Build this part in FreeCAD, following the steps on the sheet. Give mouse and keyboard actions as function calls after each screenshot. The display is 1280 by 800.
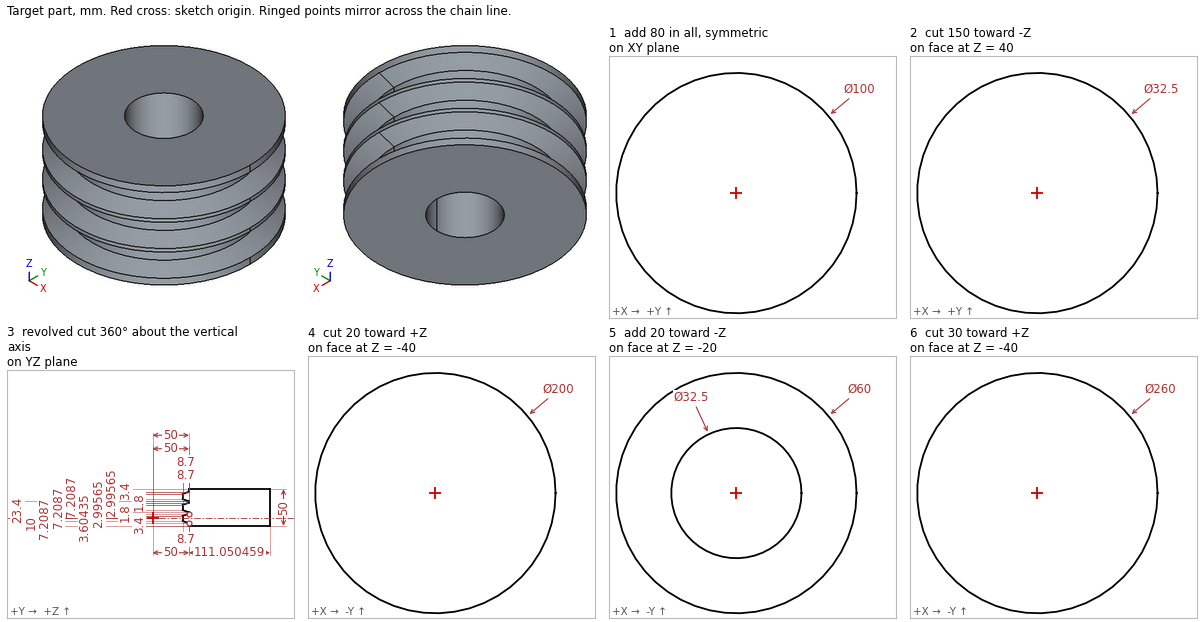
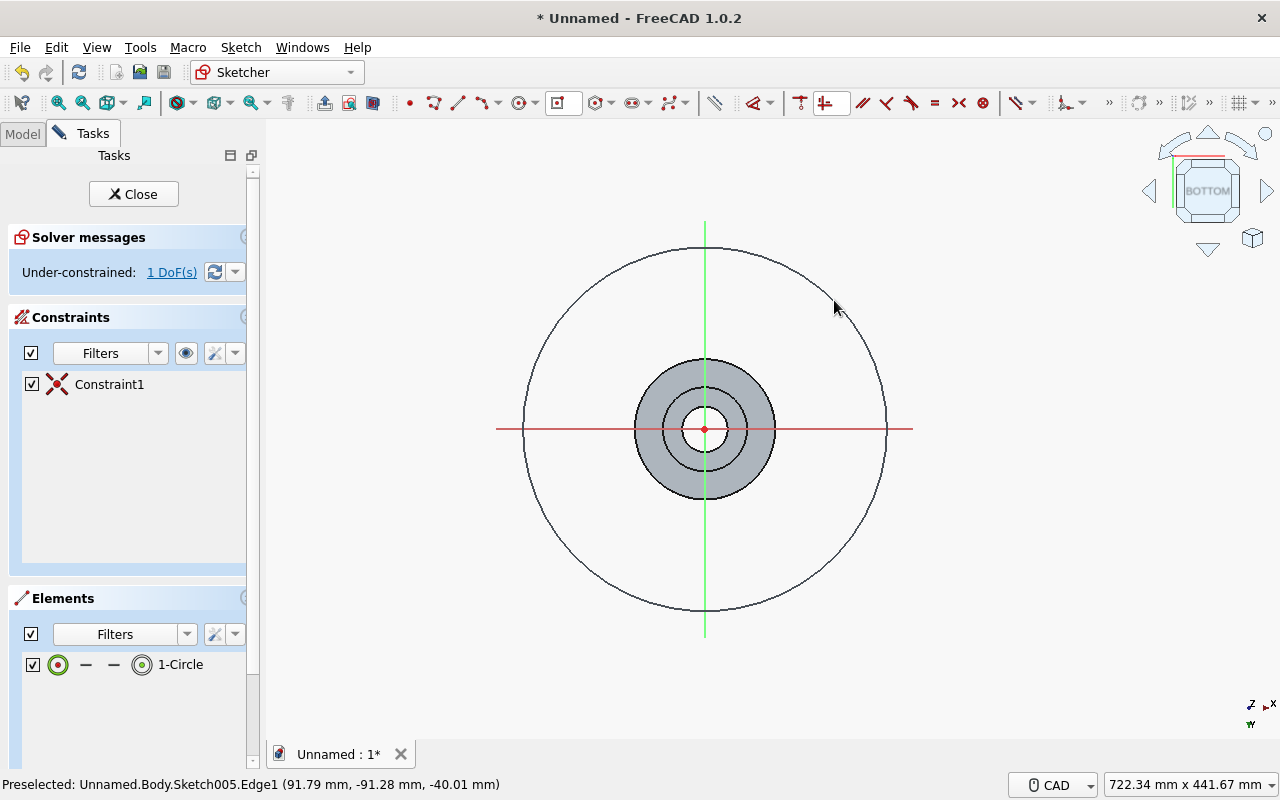
click(754, 104)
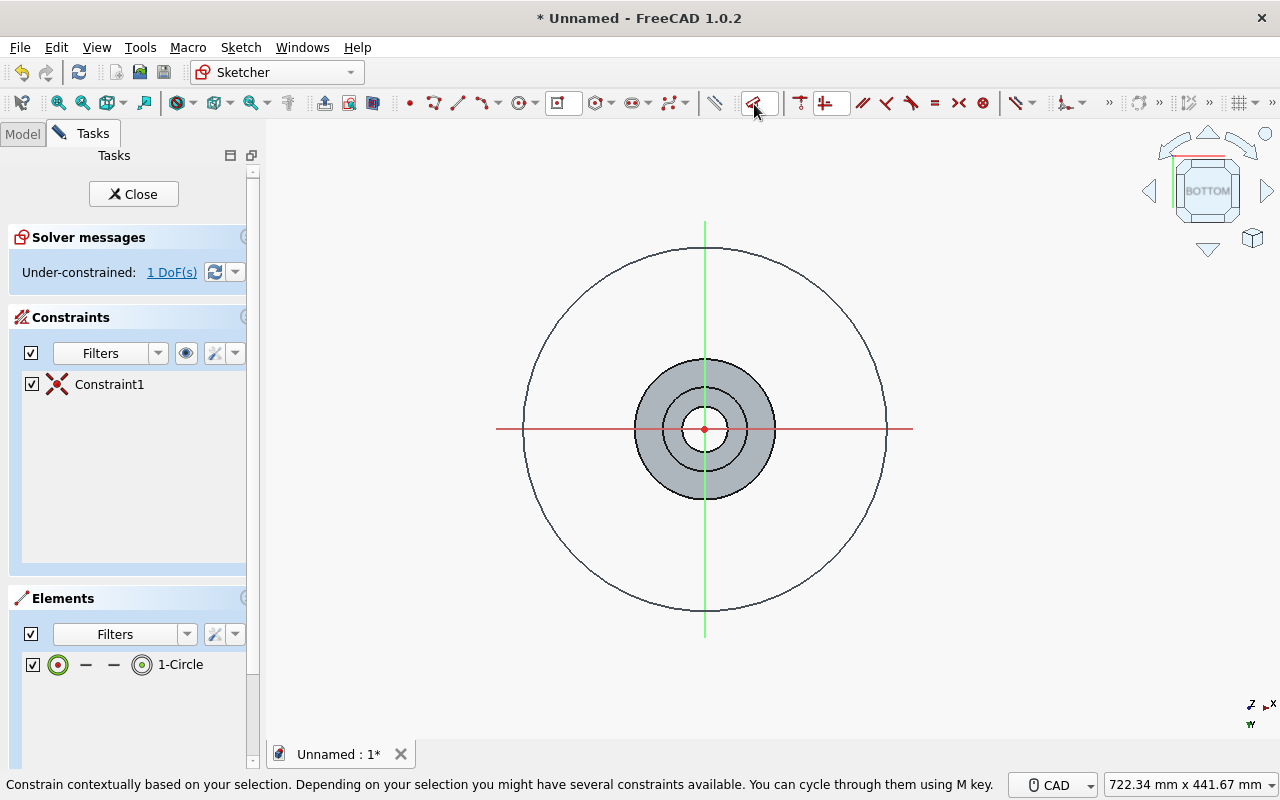
click(833, 300)
click(856, 277)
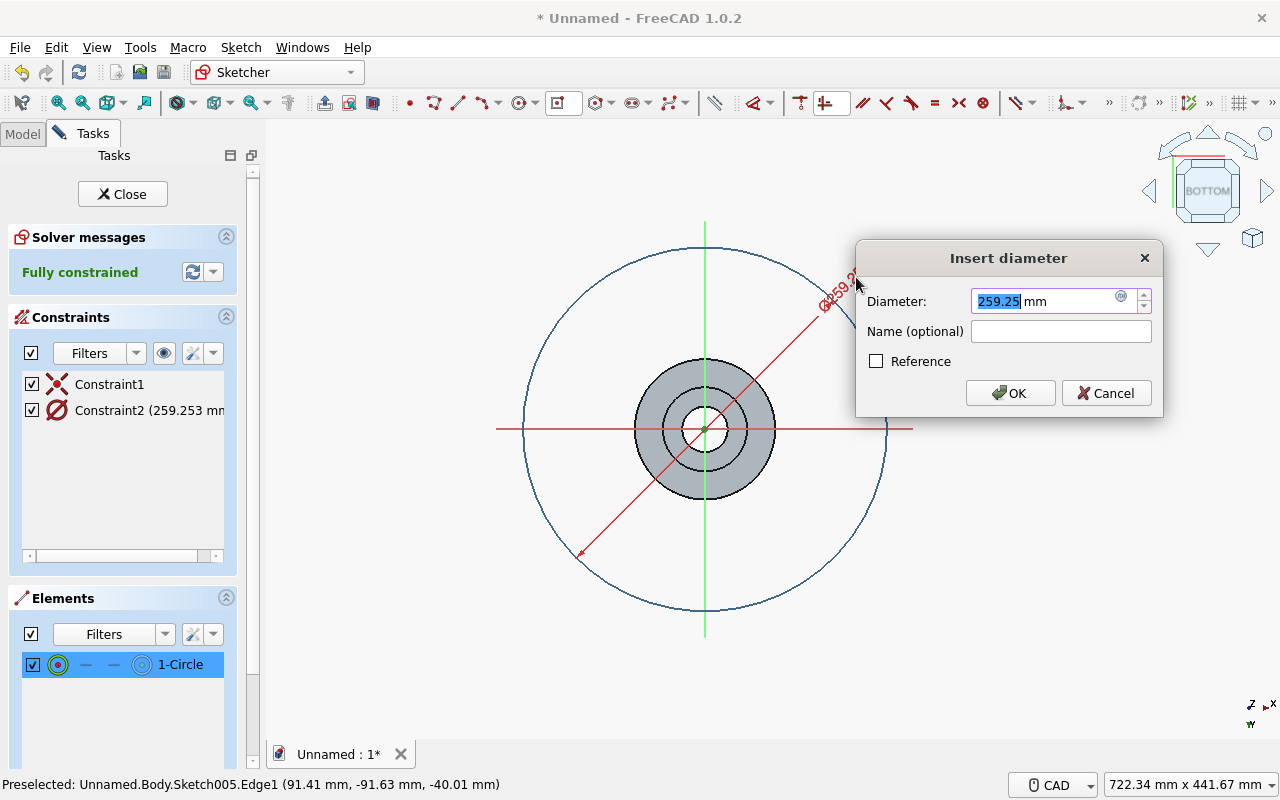
text(260)
key(Return)
key(Escape)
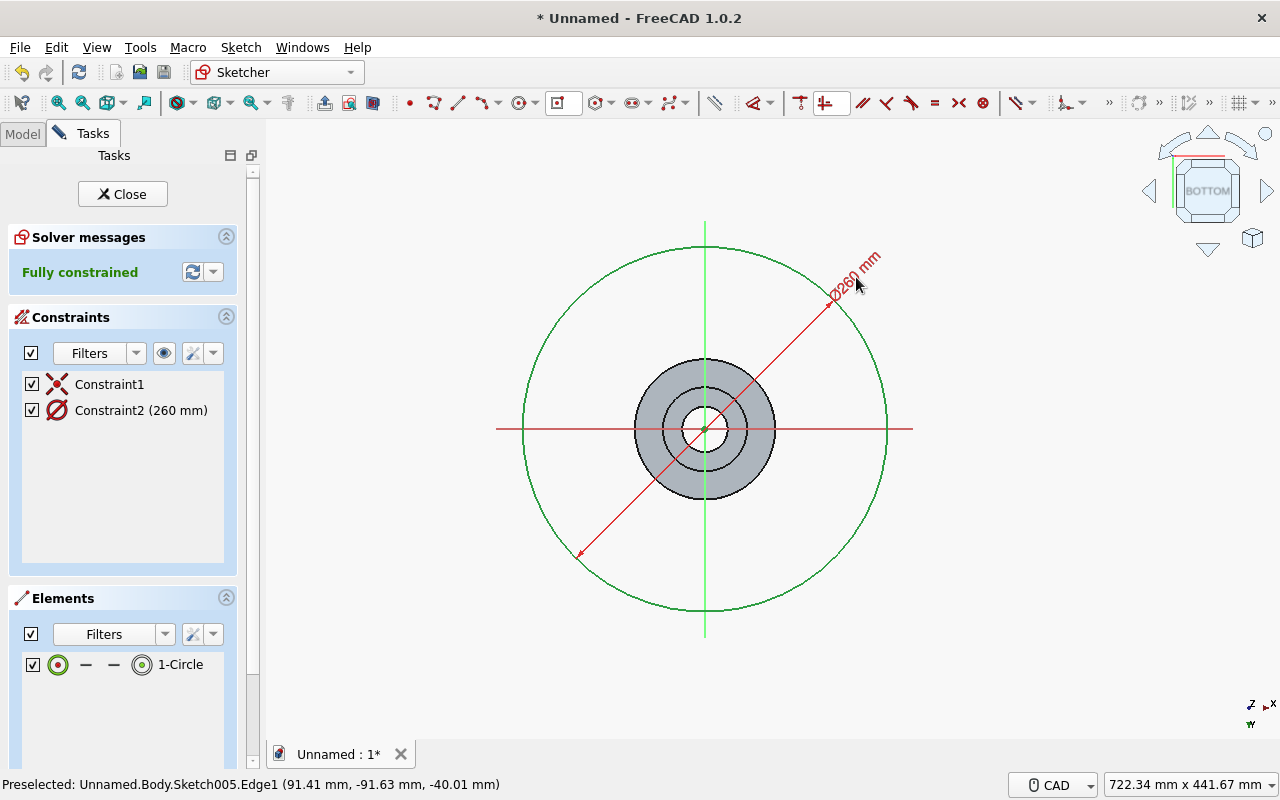
click(123, 194)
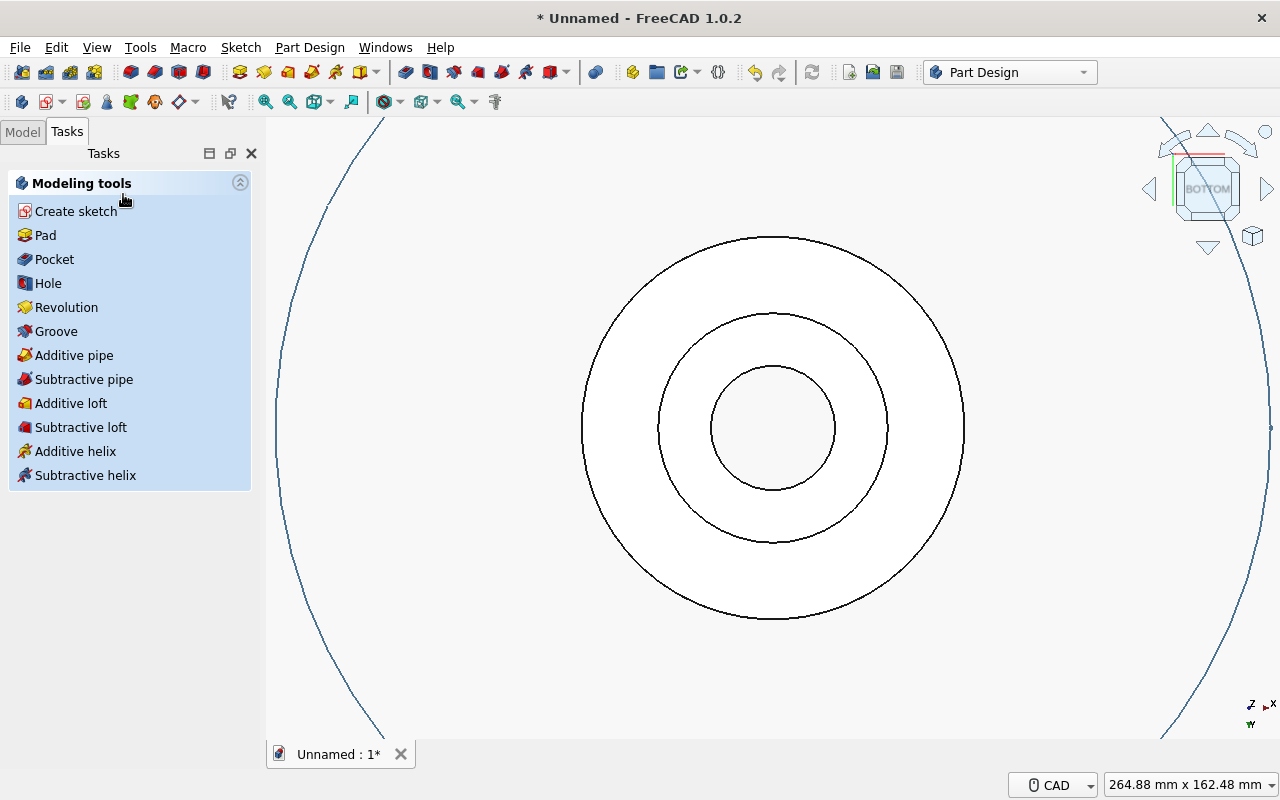
click(406, 72)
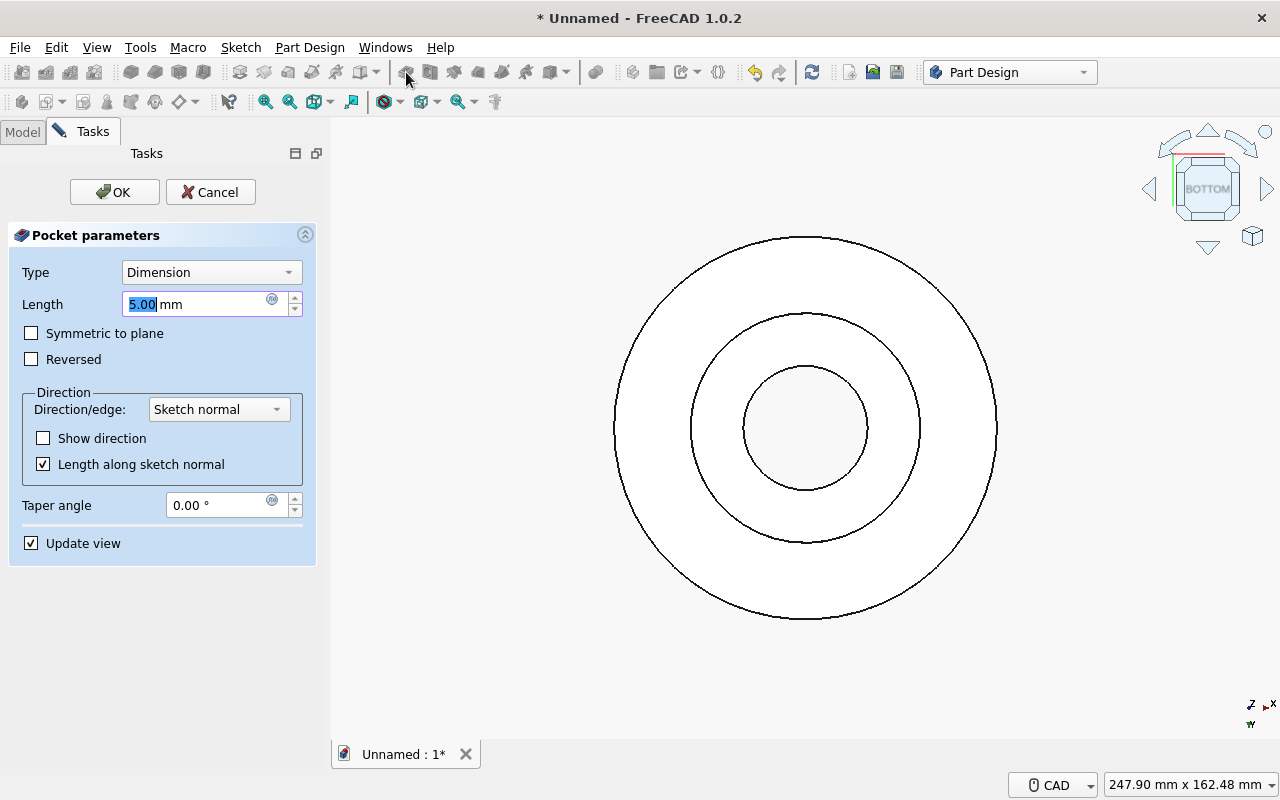
text(30)
key(Tab)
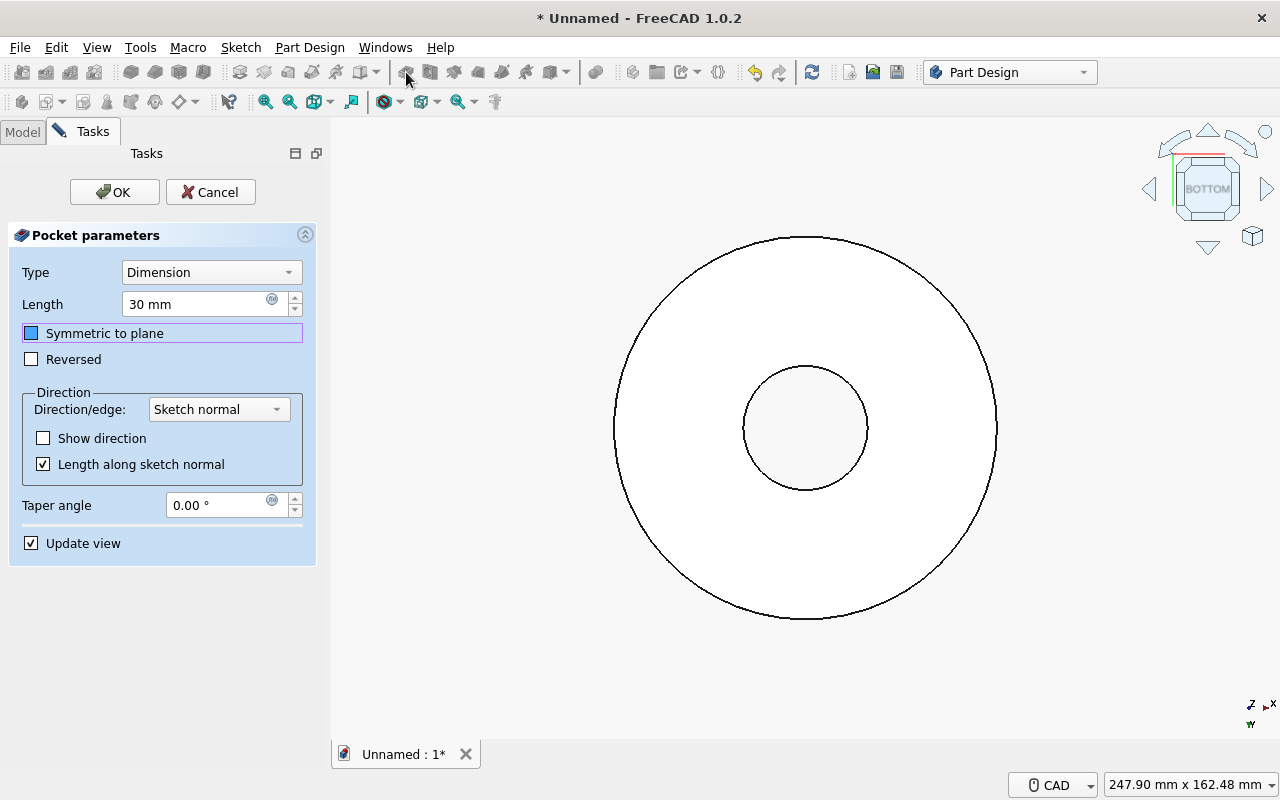
click(115, 192)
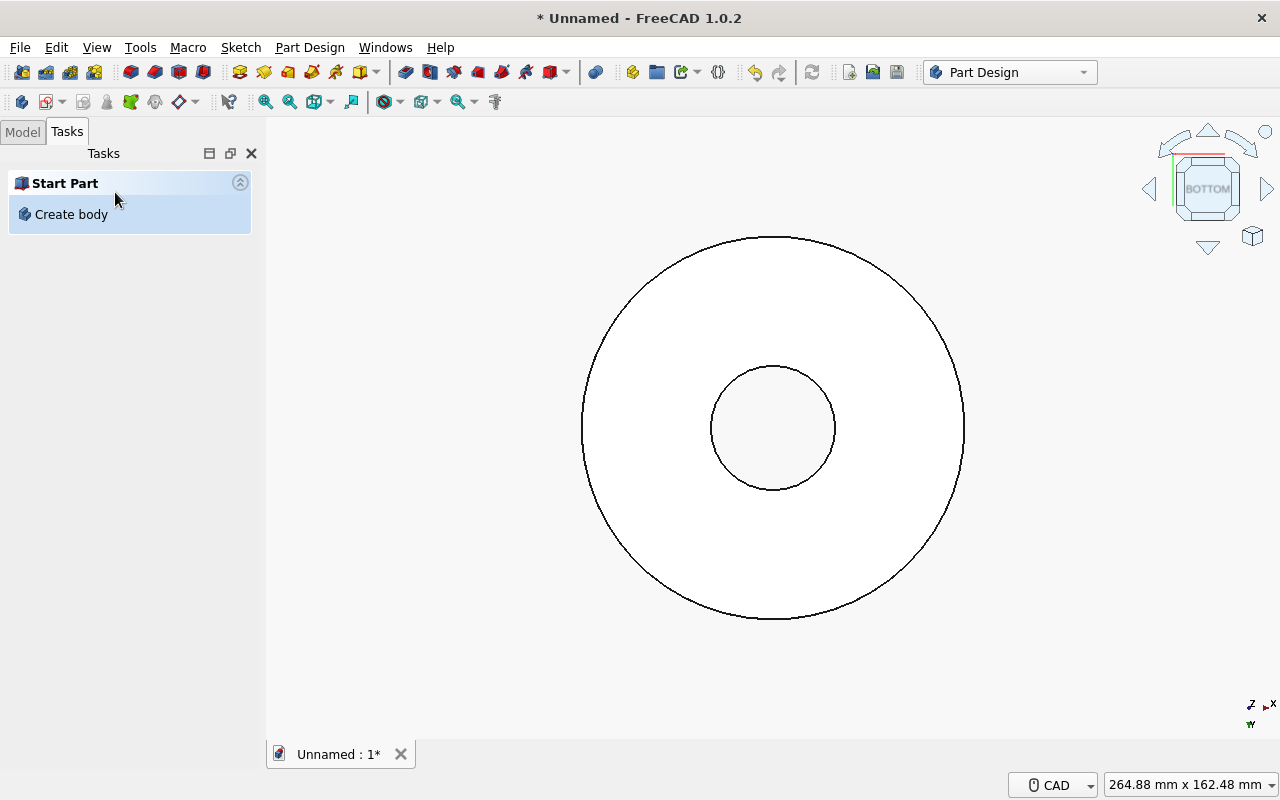
key(0)